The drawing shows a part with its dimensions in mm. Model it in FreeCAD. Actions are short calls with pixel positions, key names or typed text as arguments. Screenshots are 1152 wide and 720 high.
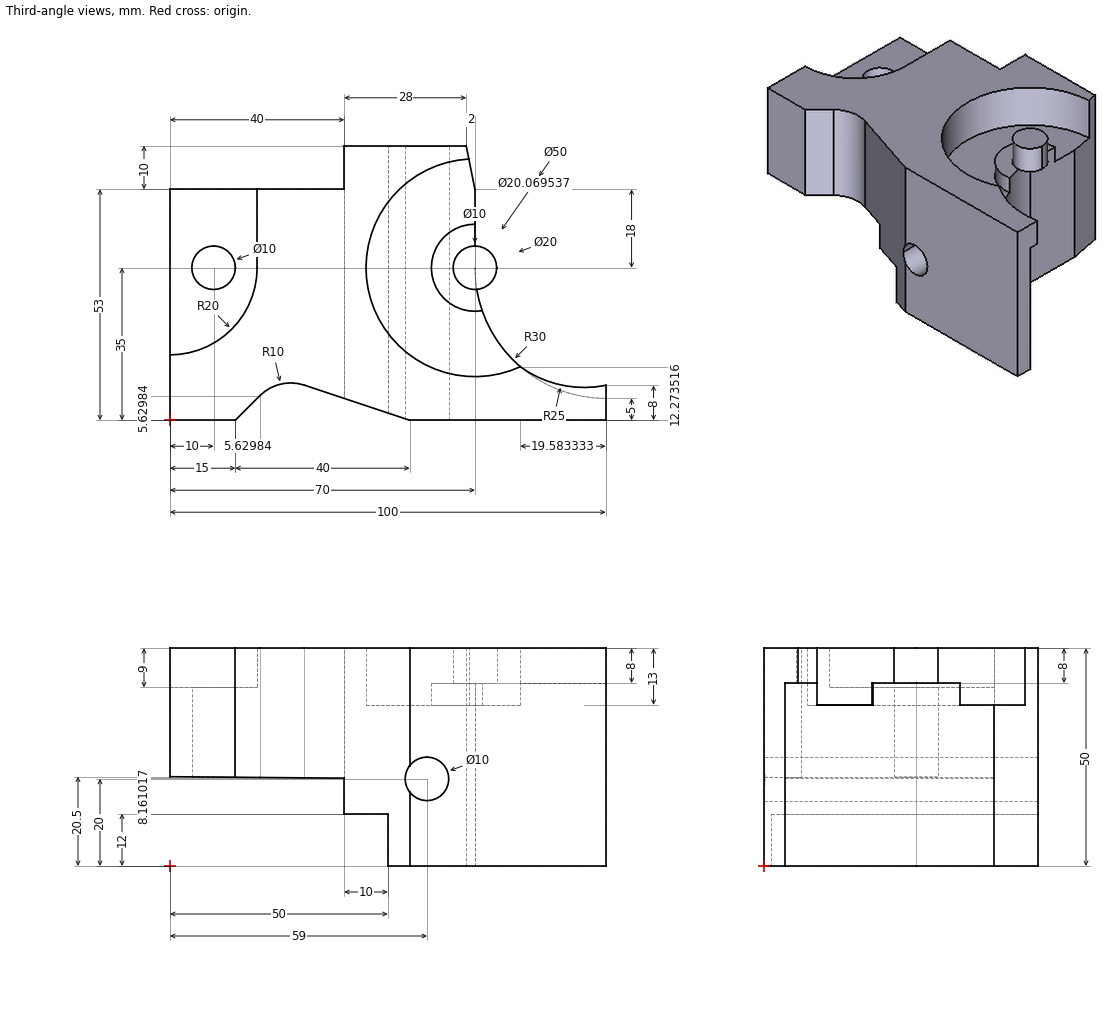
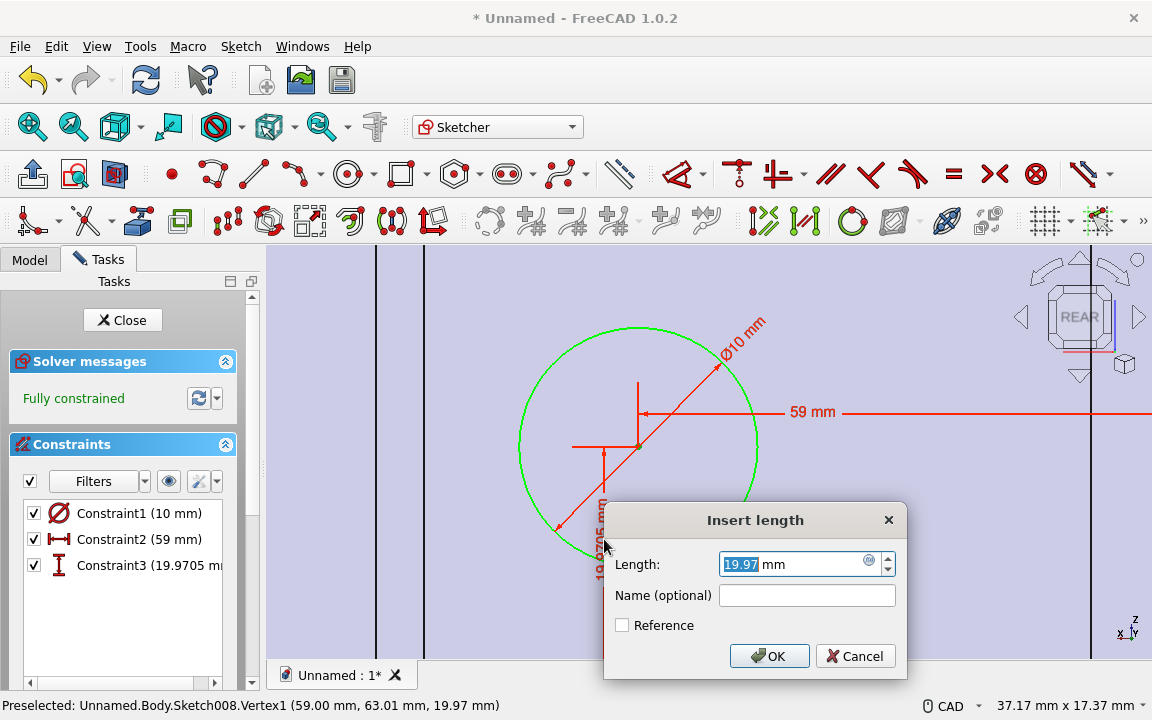
text(20)
key(Return)
key(Escape)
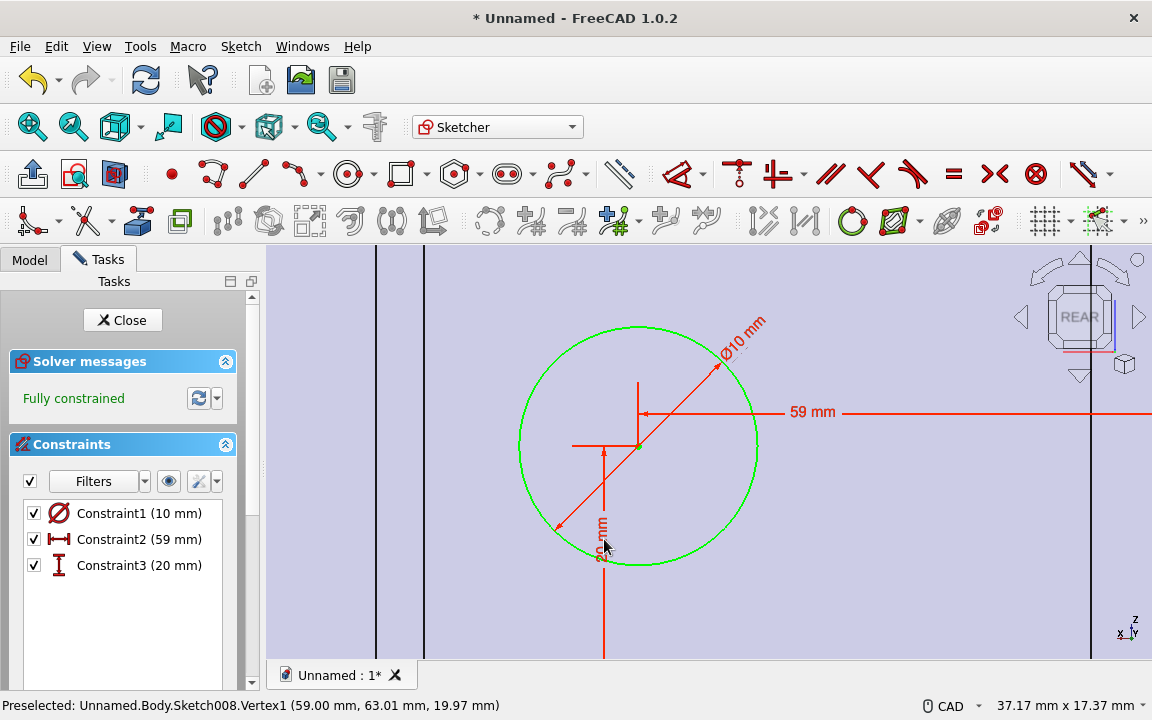
click(123, 320)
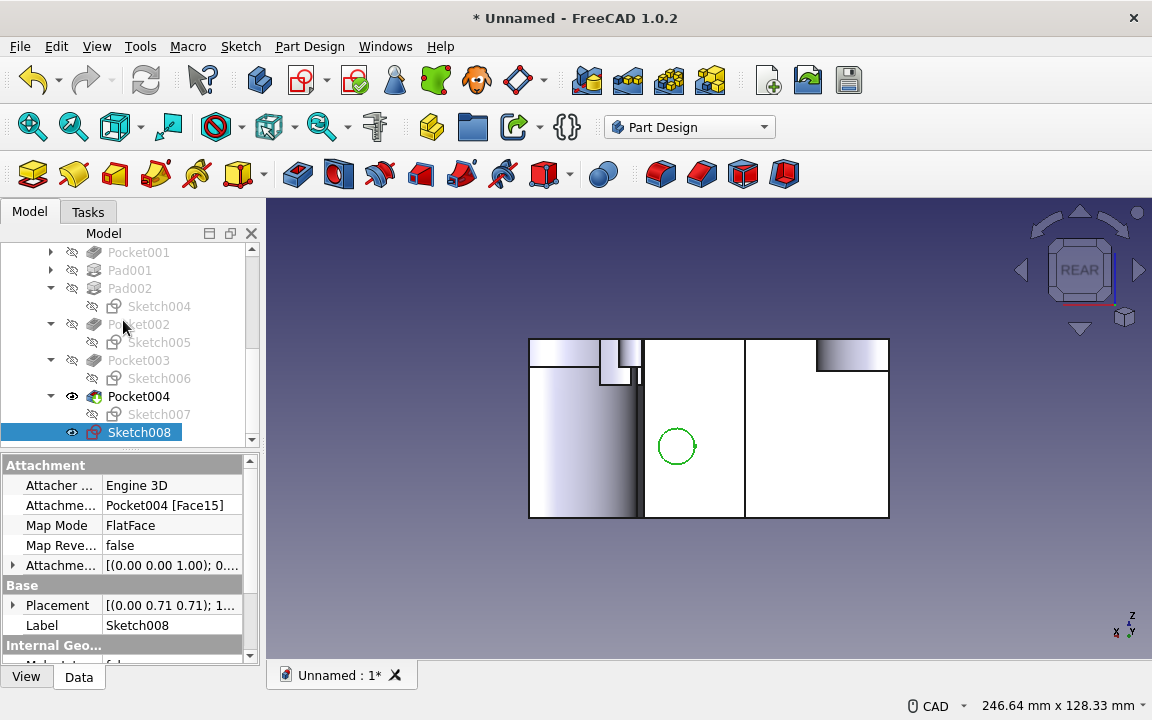
click(298, 174)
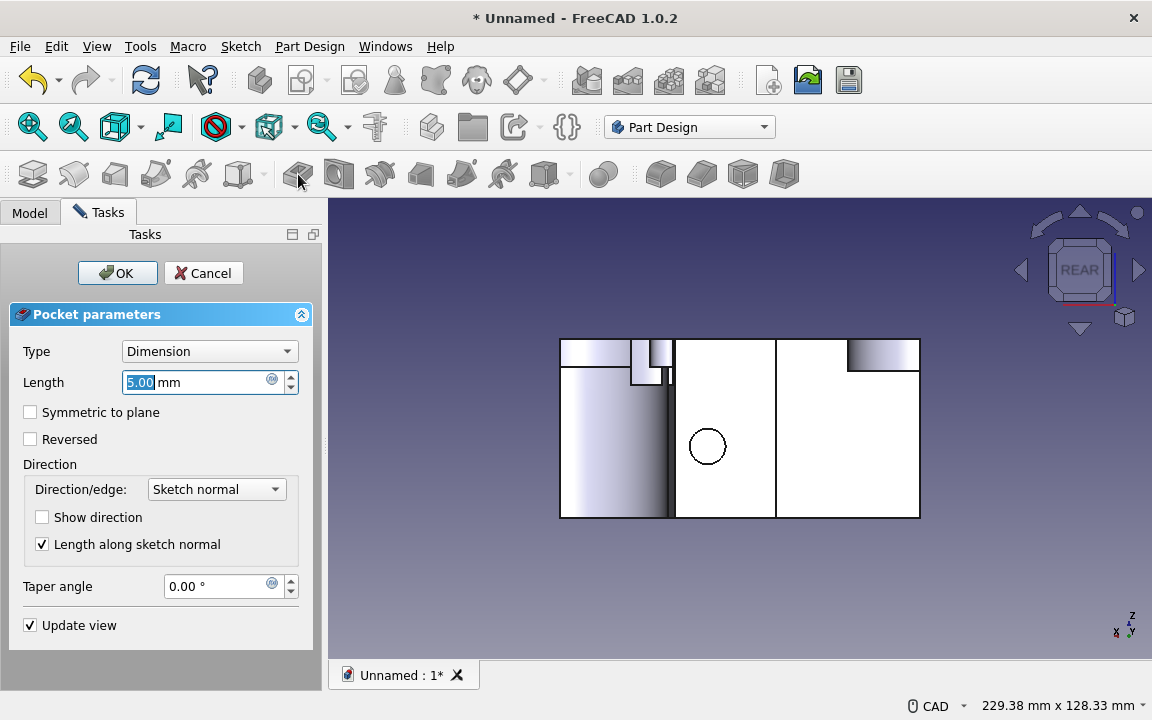
click(210, 352)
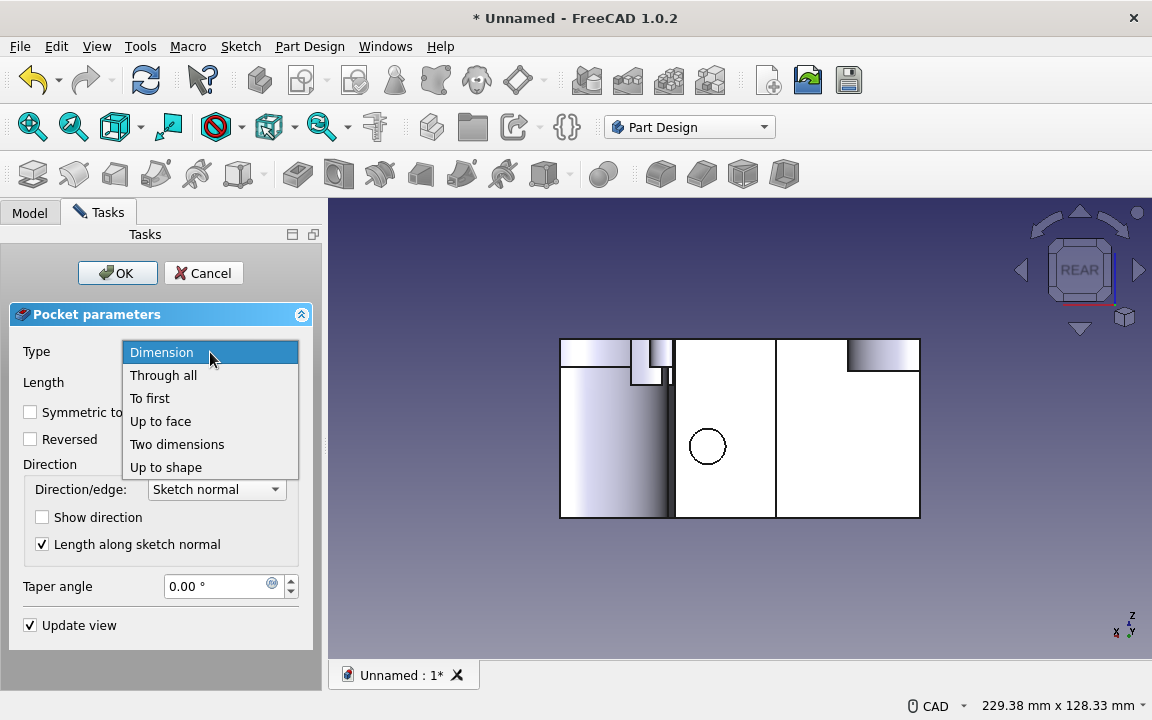
click(208, 376)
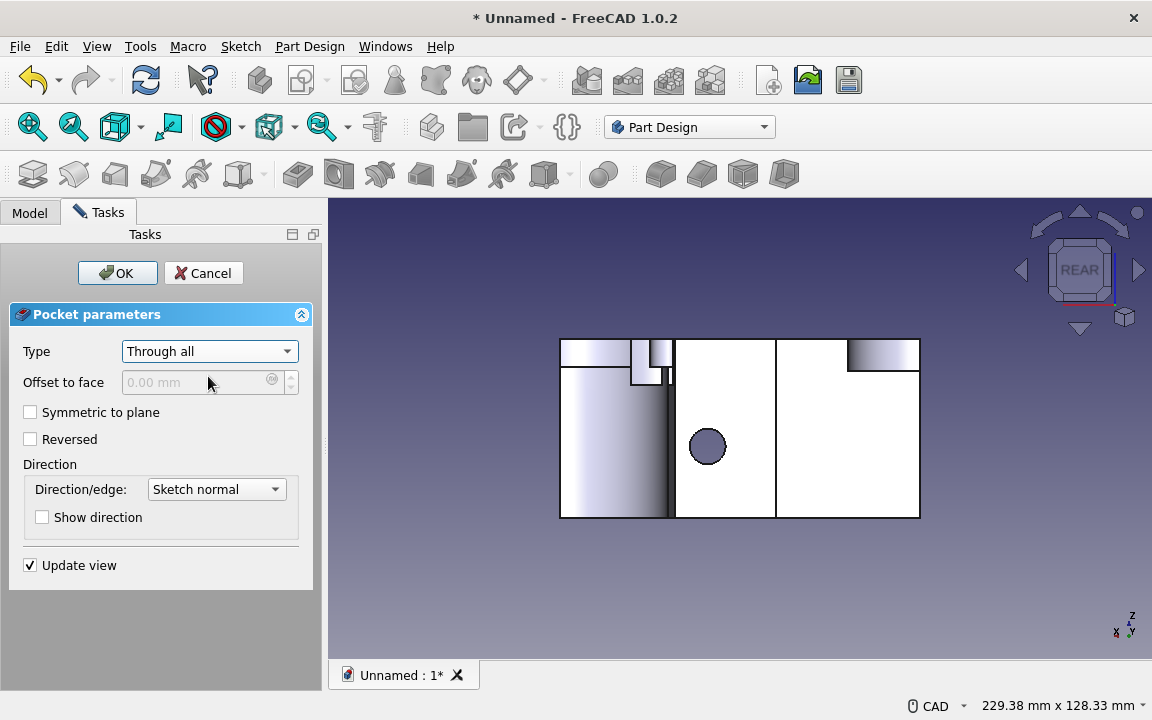
click(118, 273)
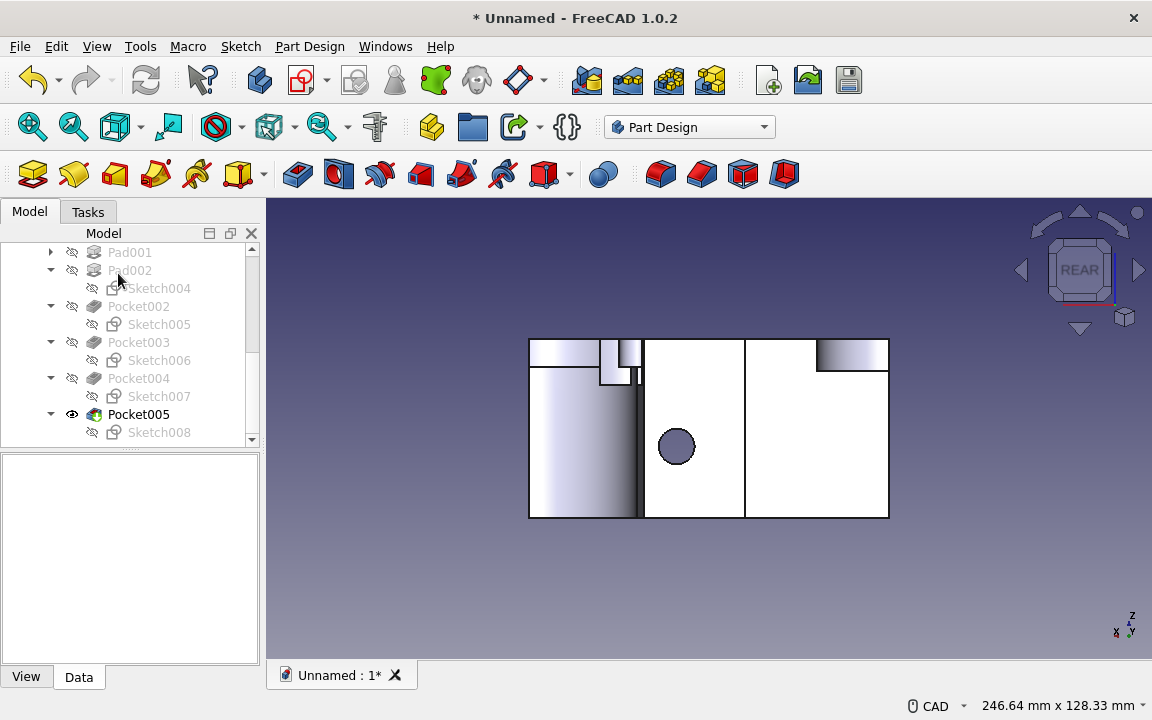
key(v)
key(f)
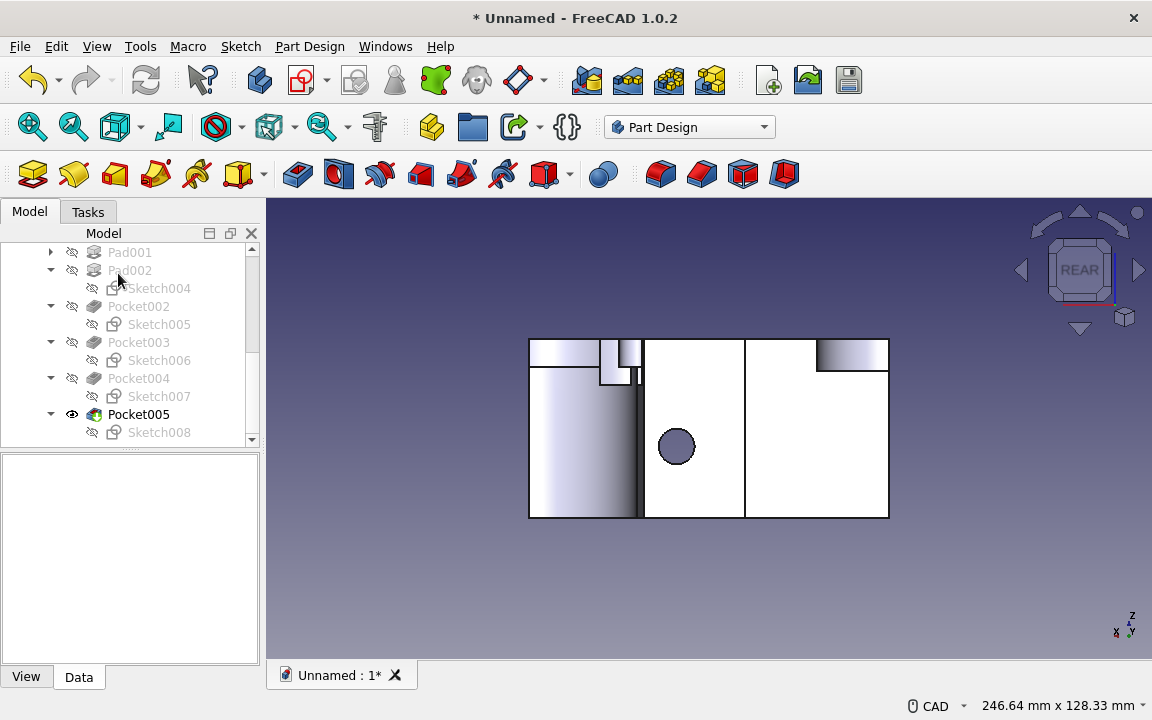
click(695, 376)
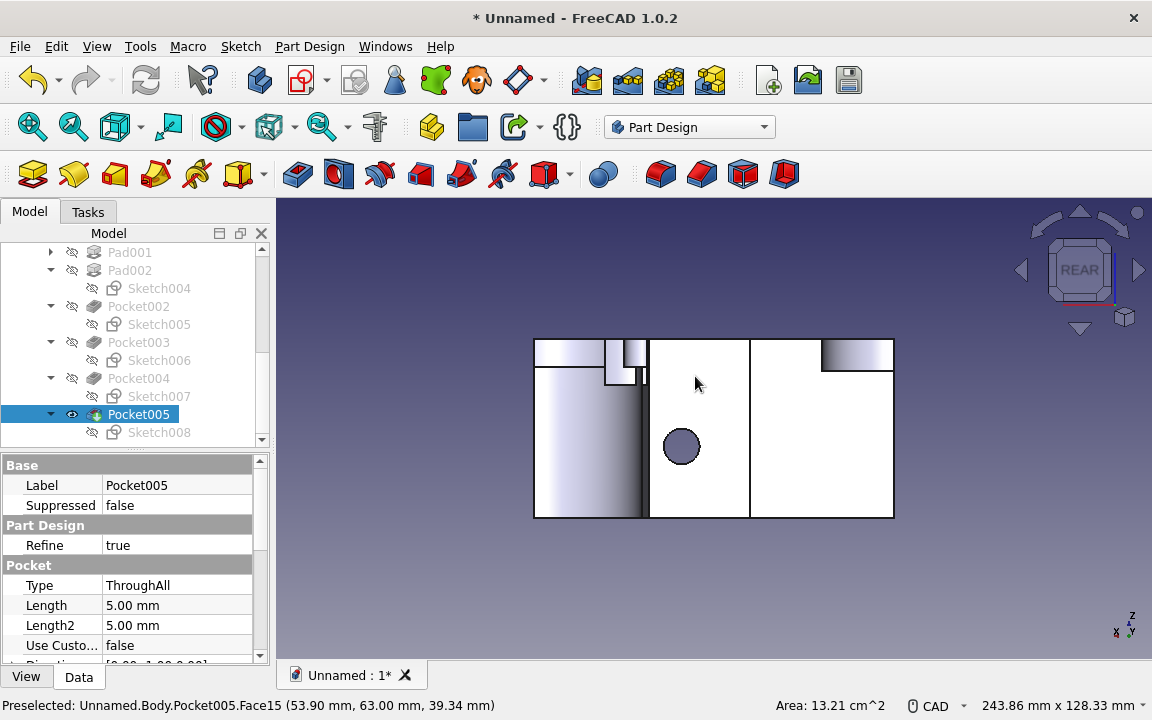
click(300, 80)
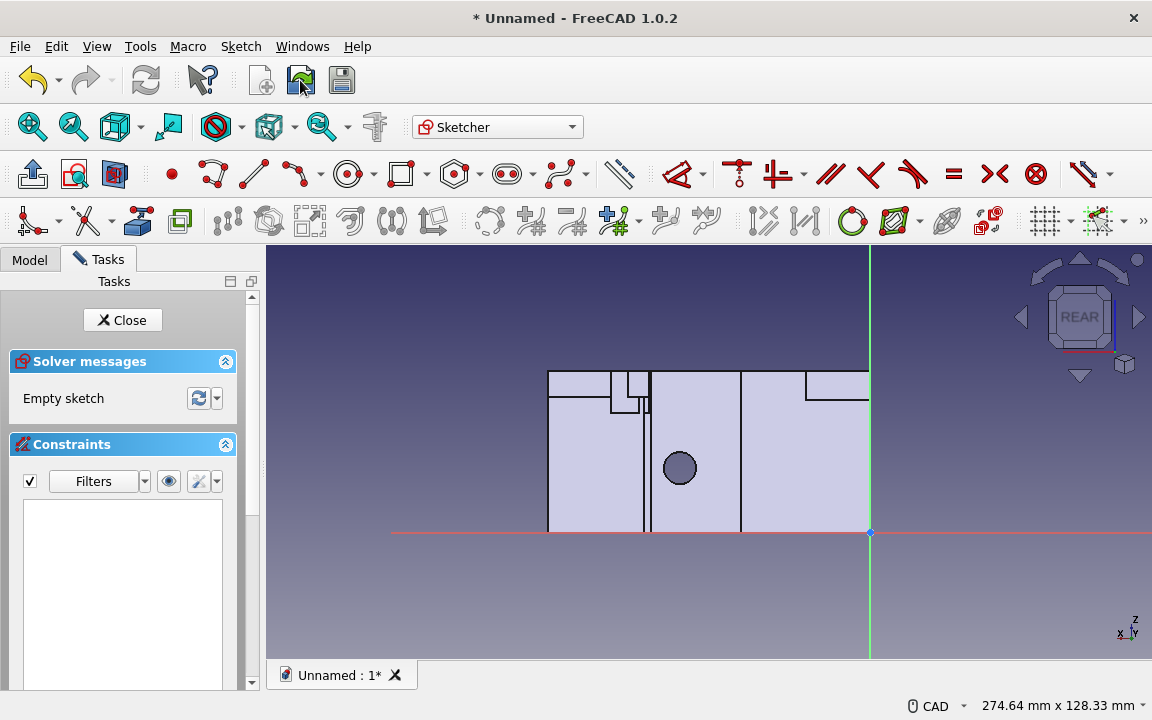
scroll(854, 520, up, 6)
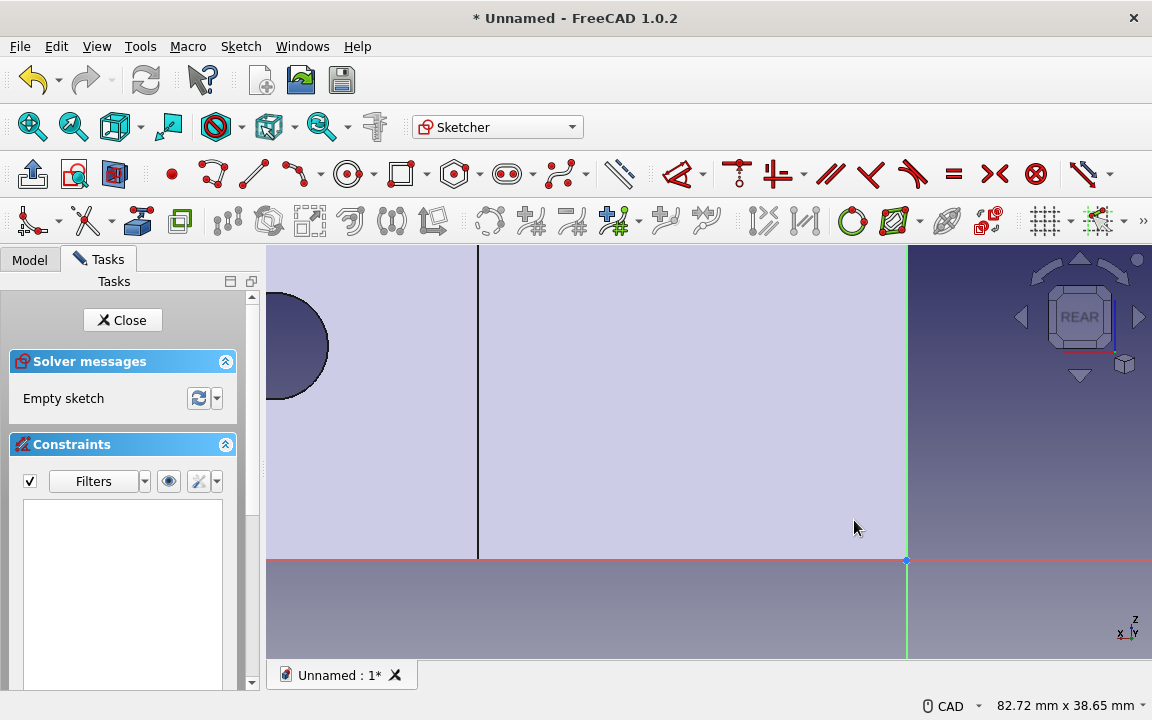
key(g)
key(m)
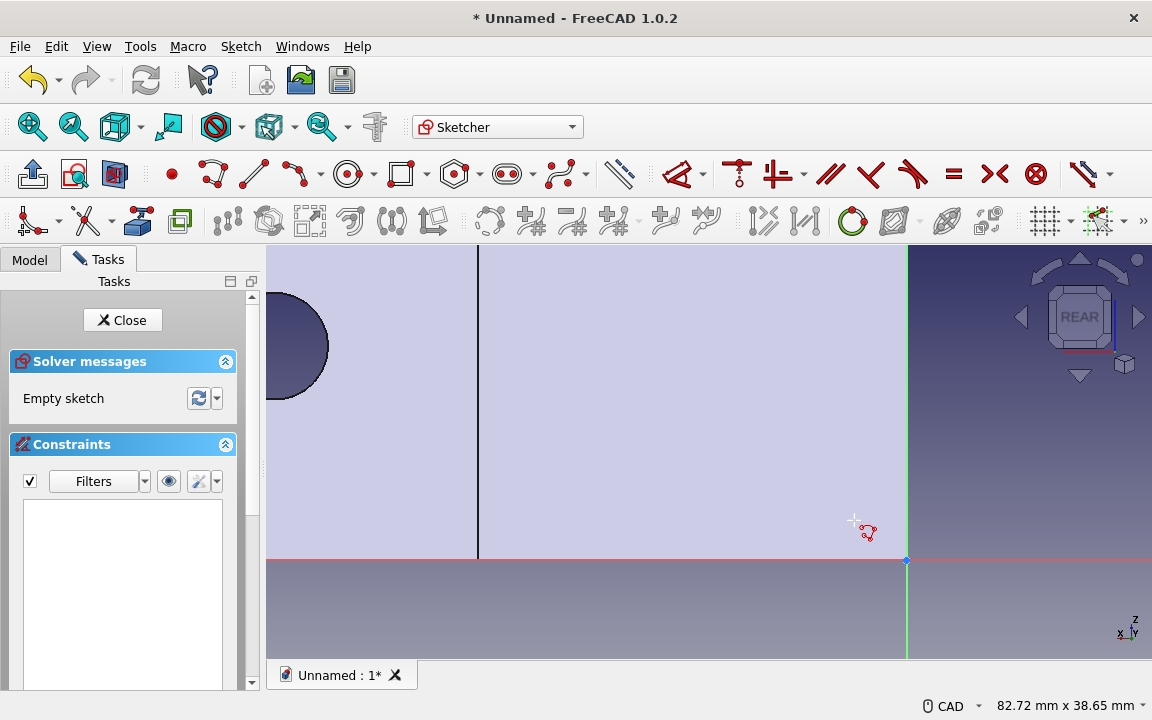
click(907, 560)
click(898, 341)
click(478, 362)
click(478, 432)
click(371, 432)
click(371, 551)
click(907, 560)
key(Escape)
key(Escape)